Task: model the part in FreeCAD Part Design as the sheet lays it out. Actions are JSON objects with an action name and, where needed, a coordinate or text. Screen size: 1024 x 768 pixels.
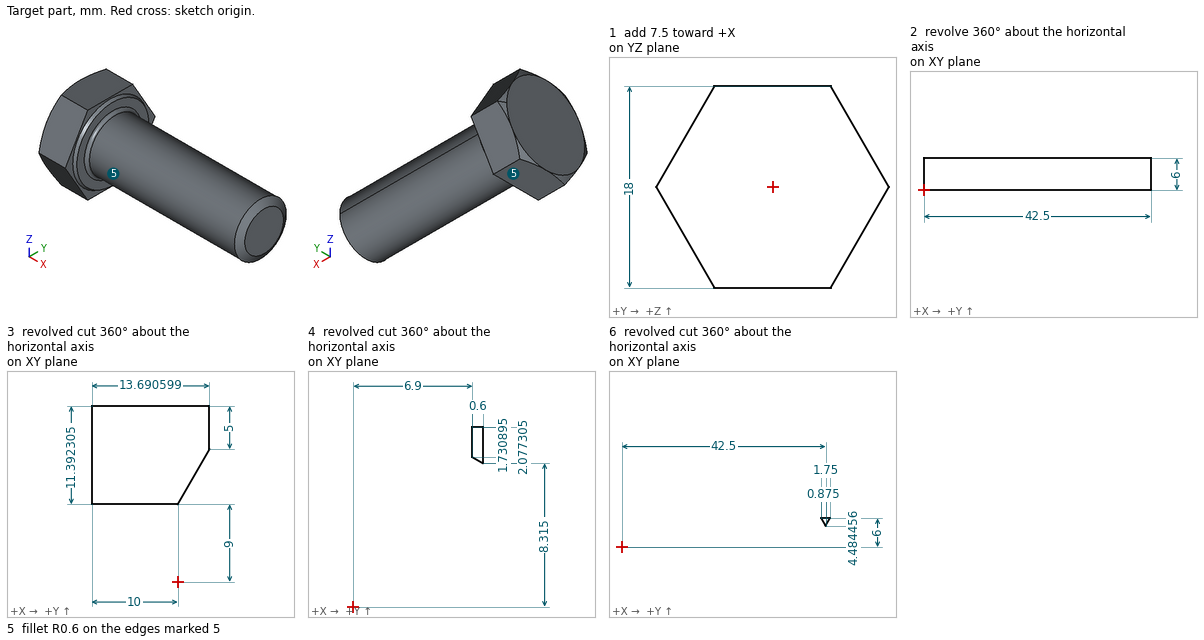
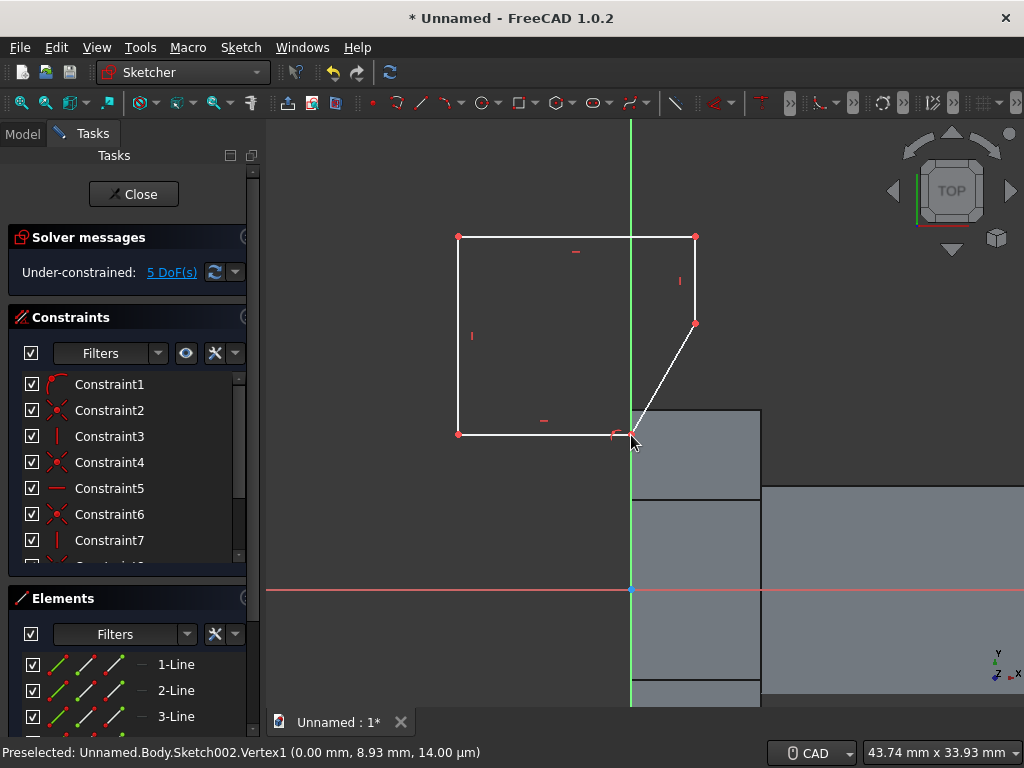
{"action": "left_click", "coordinate": [714, 104]}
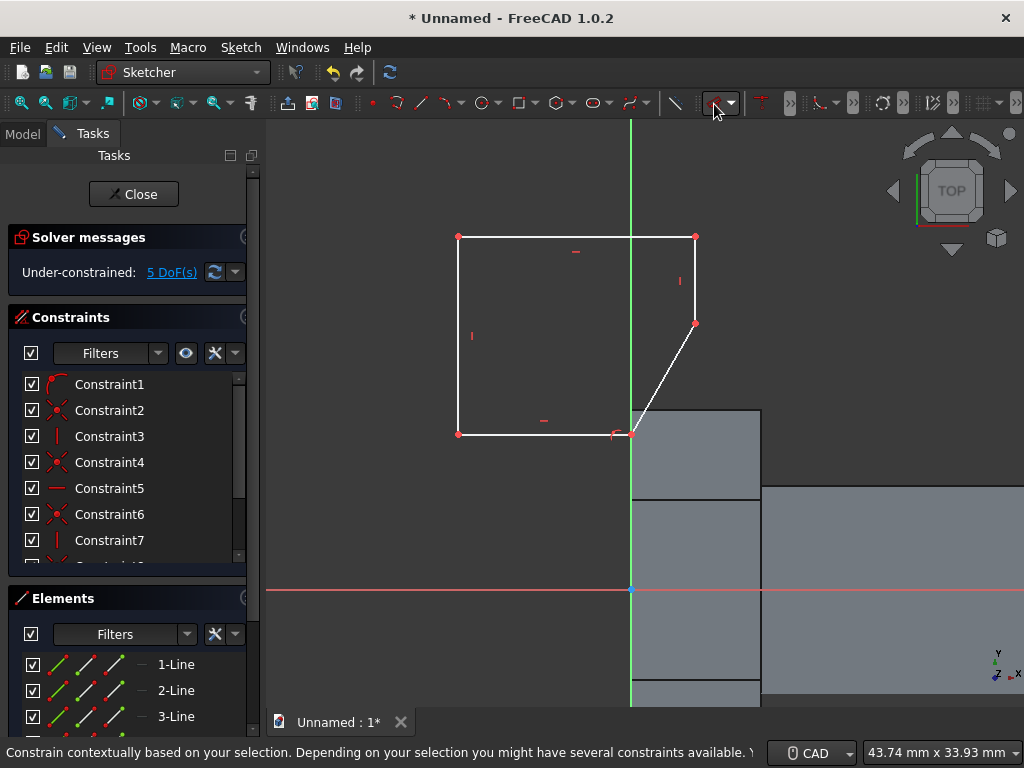
{"action": "left_click", "coordinate": [695, 298]}
{"action": "left_click", "coordinate": [729, 280]}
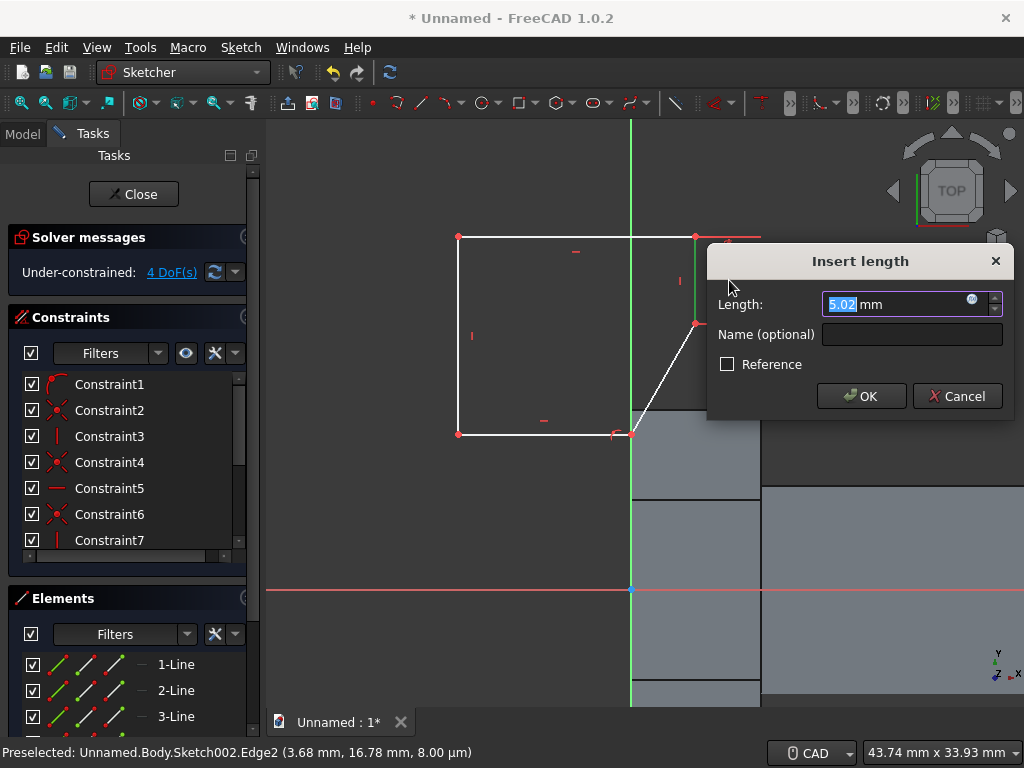
{"action": "type", "text": "5"}
{"action": "key", "text": "Return"}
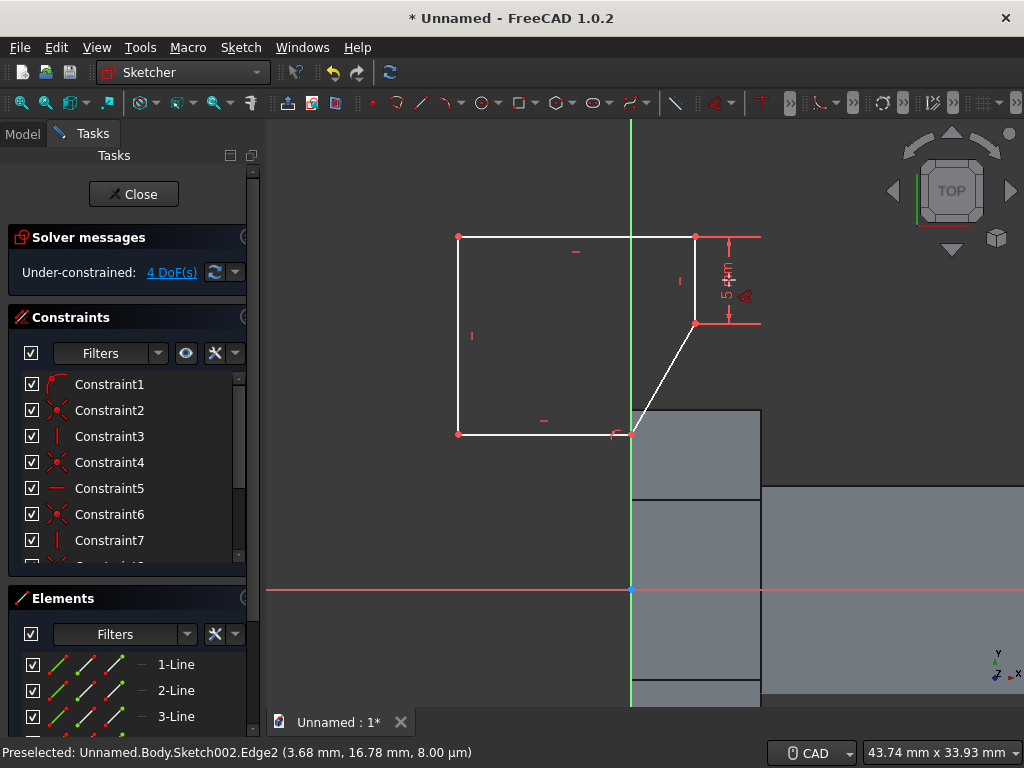
{"action": "left_click", "coordinate": [510, 435]}
{"action": "left_click", "coordinate": [545, 469]}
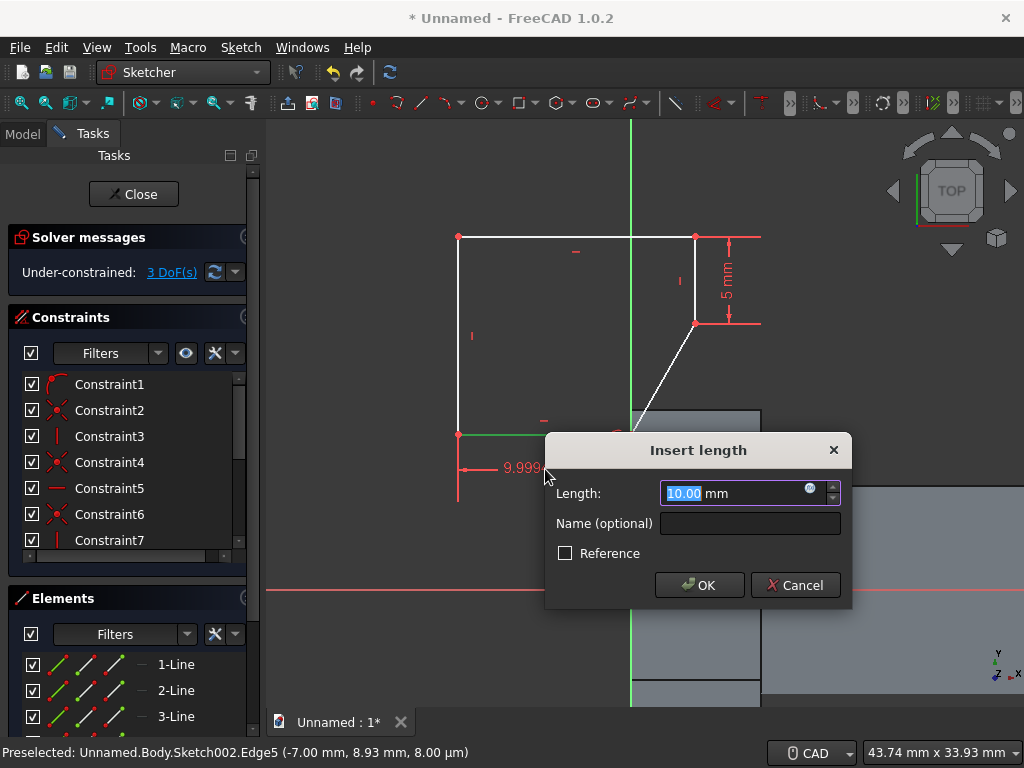
{"action": "type", "text": "10"}
{"action": "key", "text": "Return"}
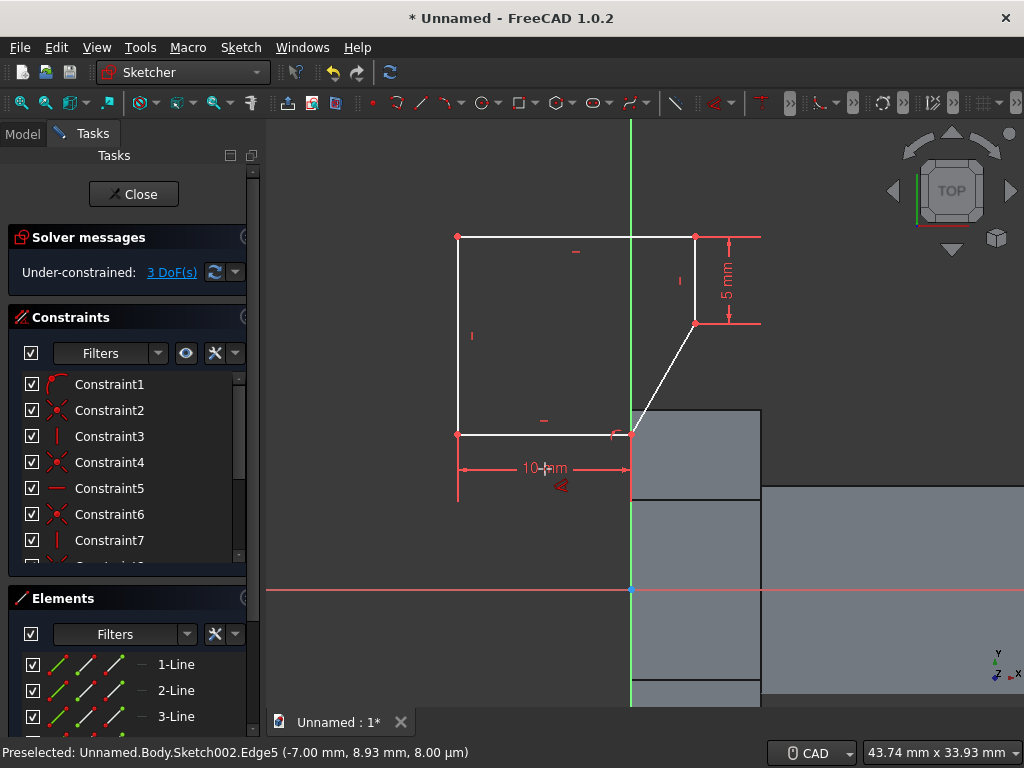
{"action": "left_click", "coordinate": [631, 435]}
{"action": "left_click", "coordinate": [665, 512]}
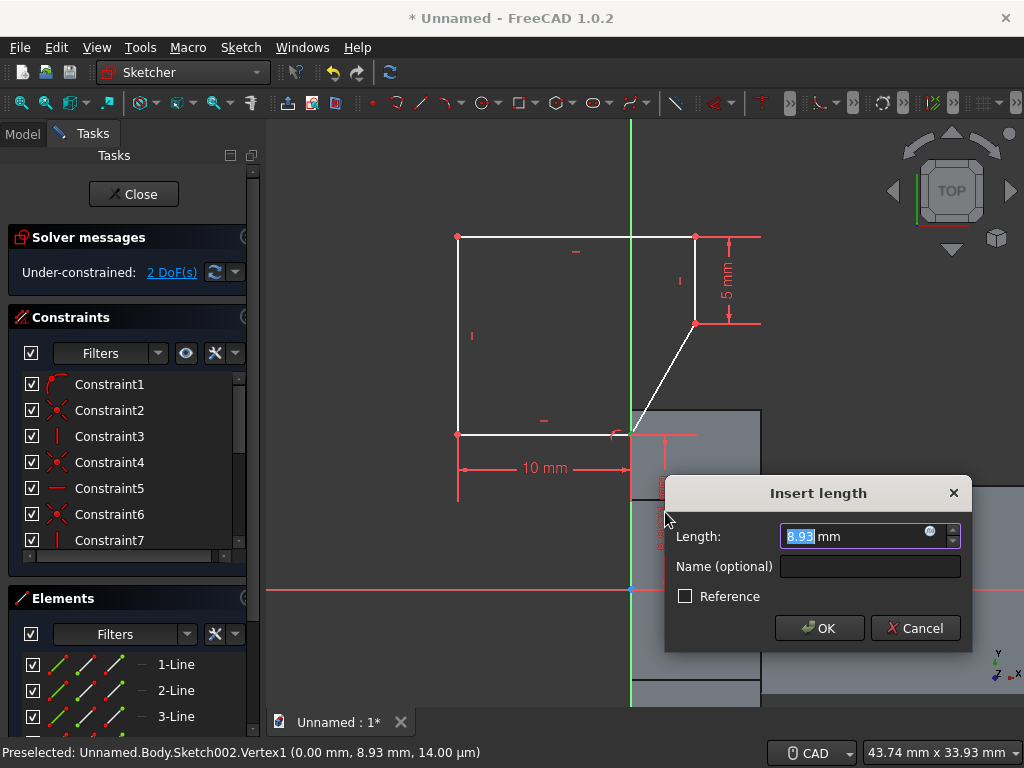
{"action": "type", "text": "9"}
{"action": "key", "text": "Return"}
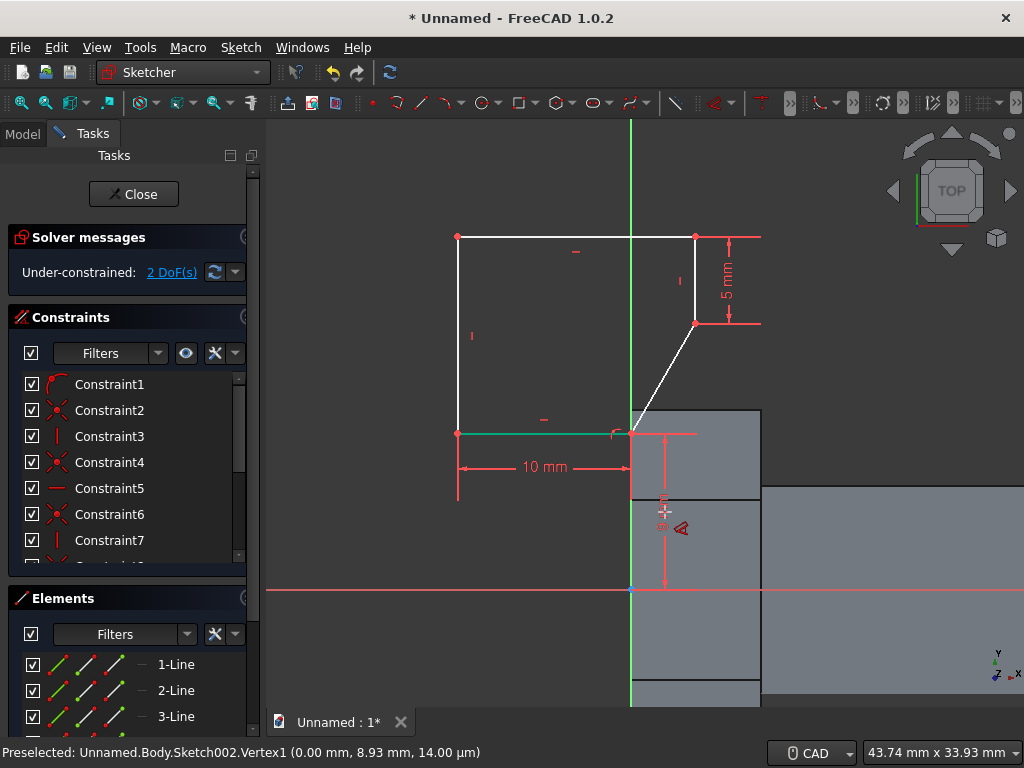
{"action": "left_click", "coordinate": [529, 237]}
{"action": "left_click", "coordinate": [576, 203]}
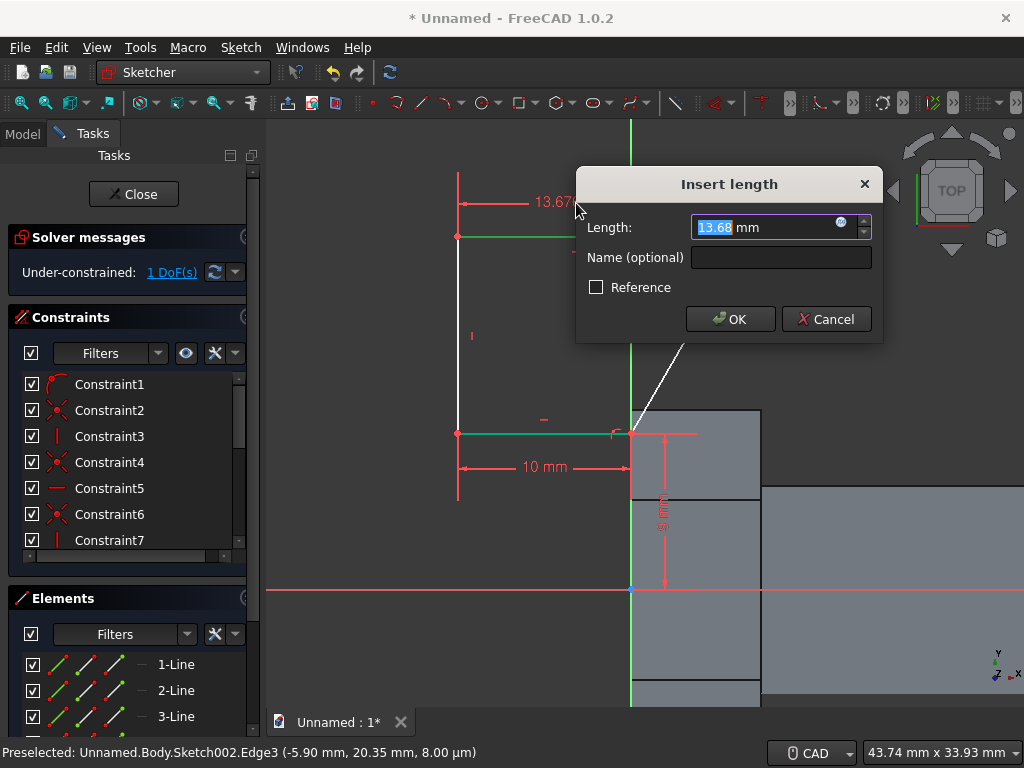
{"action": "type", "text": "13.690599"}
{"action": "key", "text": "Return"}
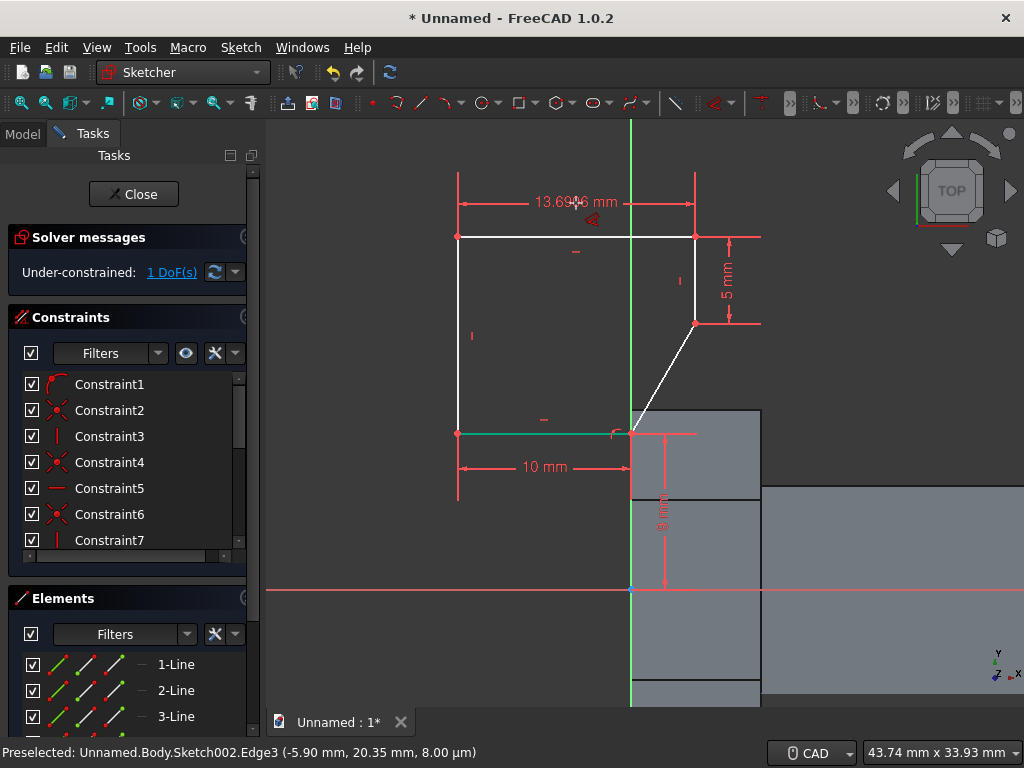
{"action": "left_click", "coordinate": [458, 296]}
{"action": "left_click", "coordinate": [424, 335]}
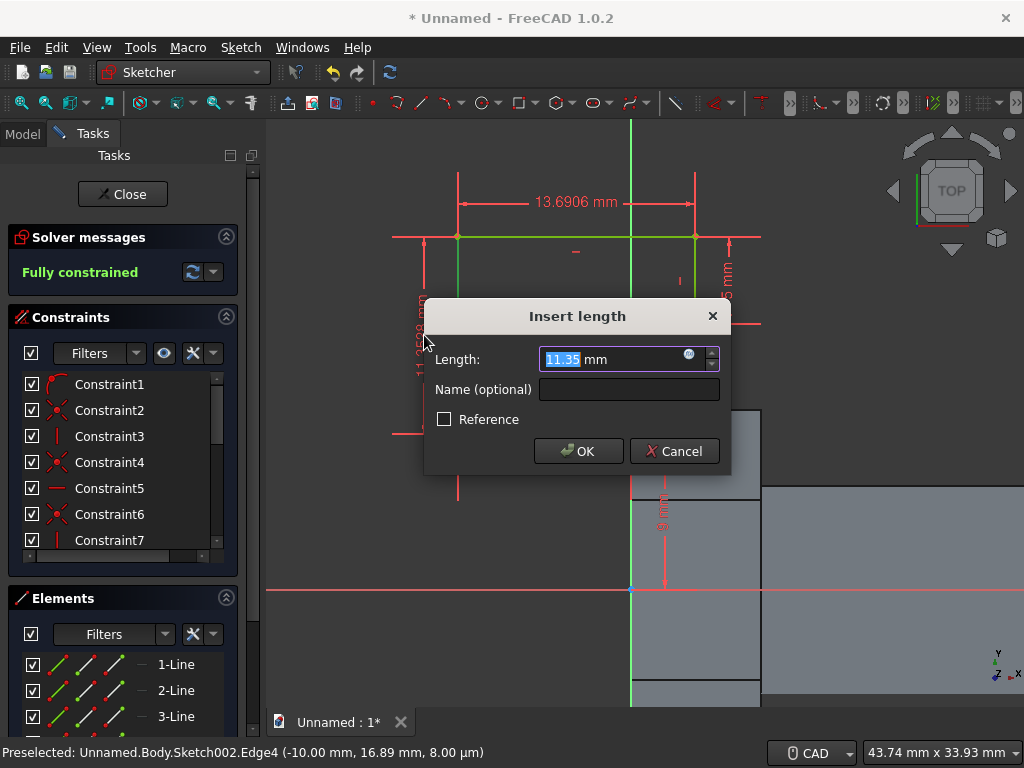
{"action": "type", "text": "11.392305"}
{"action": "key", "text": "Return"}
{"action": "key", "text": "Escape"}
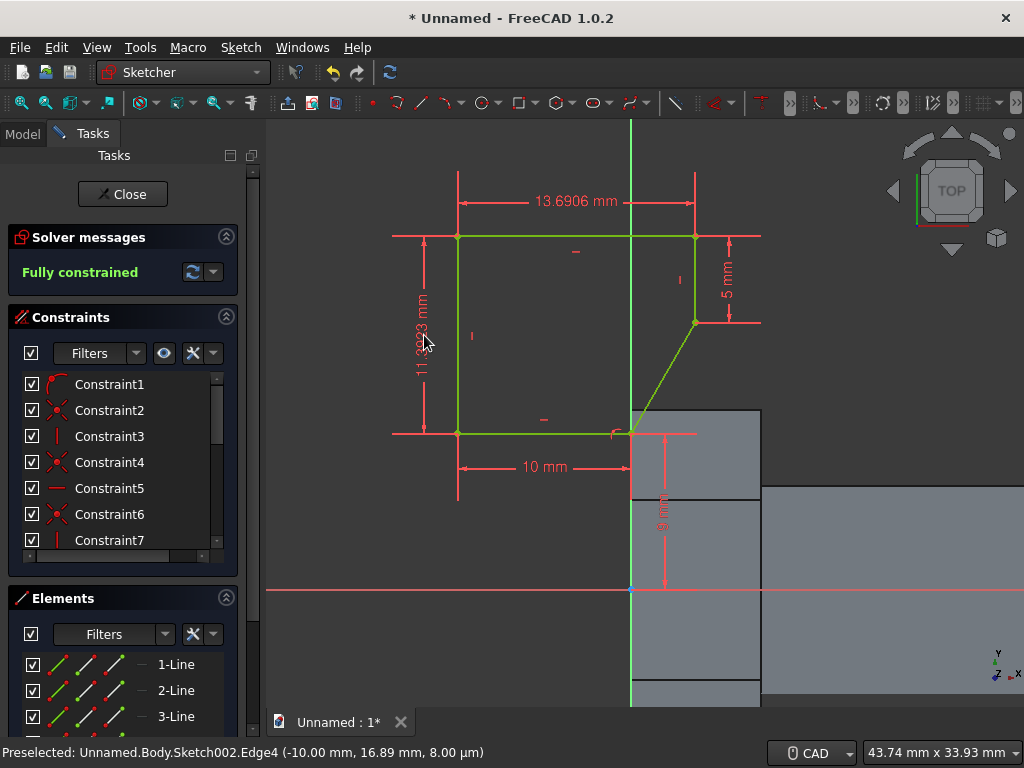
{"action": "left_click", "coordinate": [123, 194]}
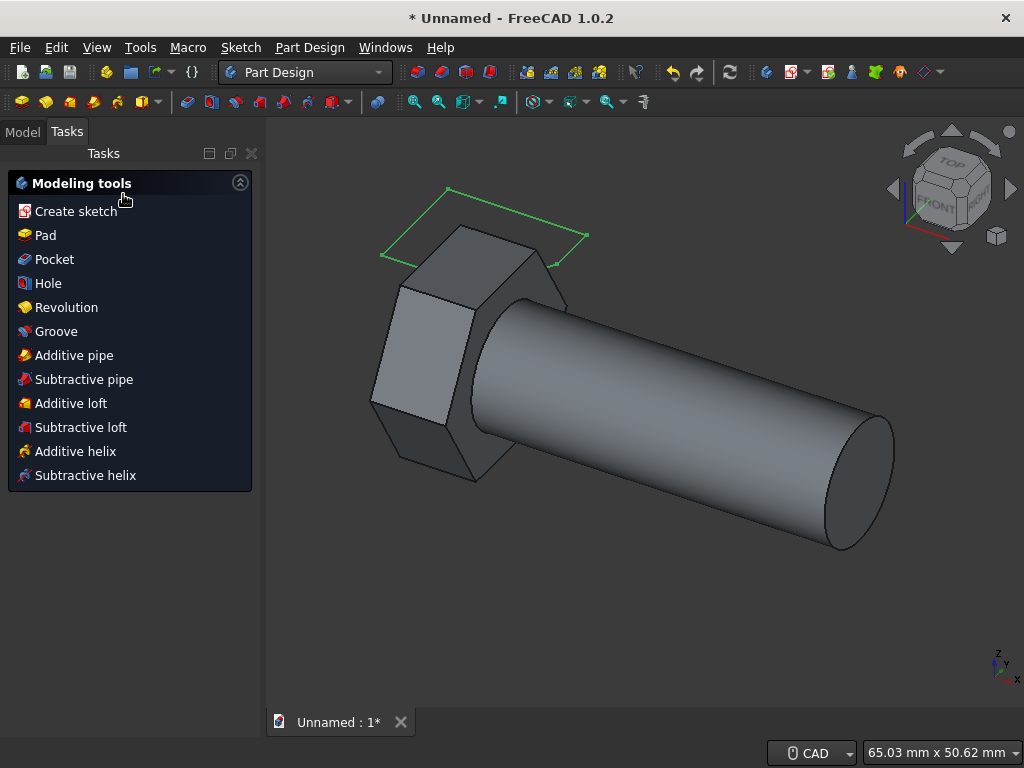
{"action": "left_click", "coordinate": [236, 102]}